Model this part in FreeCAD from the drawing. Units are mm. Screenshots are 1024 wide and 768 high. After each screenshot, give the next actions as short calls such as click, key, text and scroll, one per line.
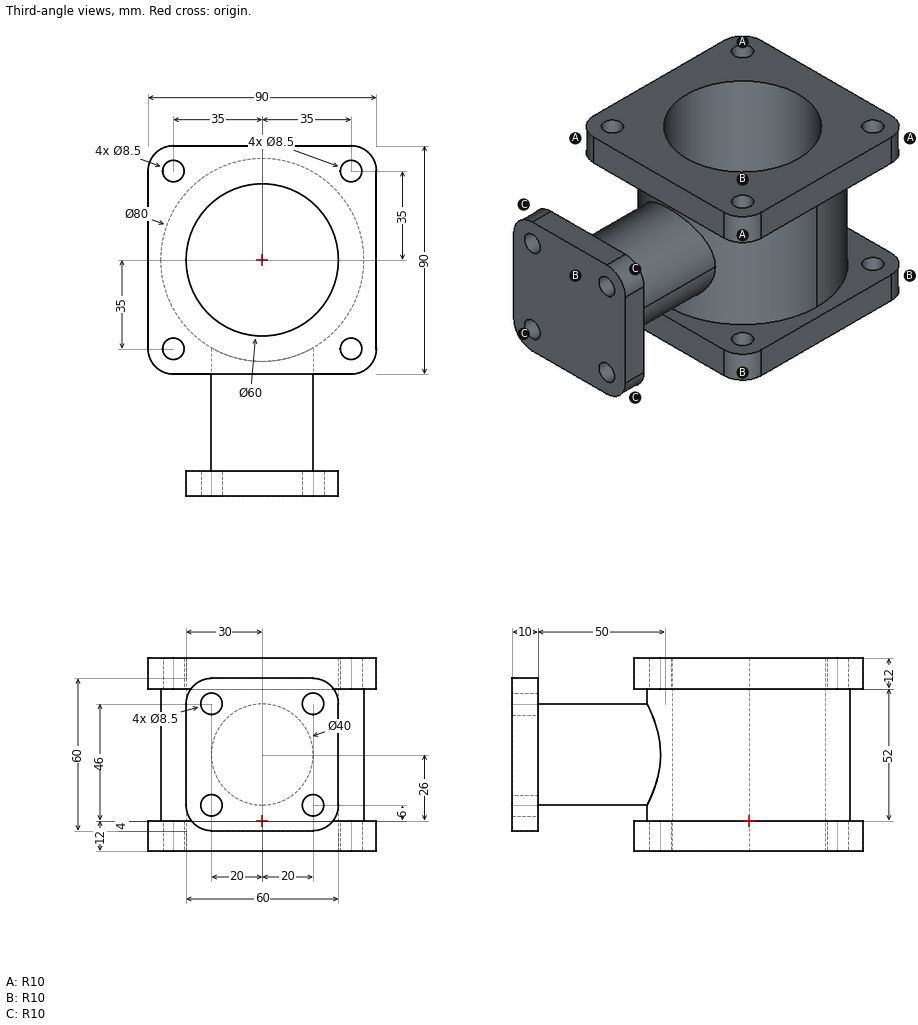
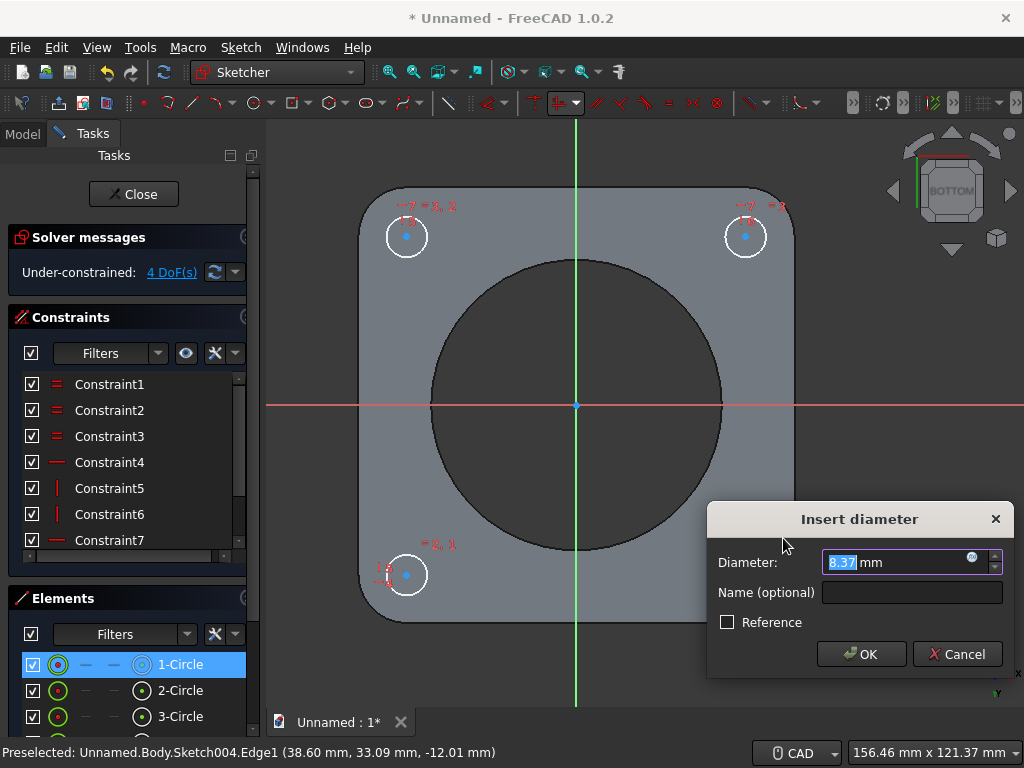
text(8.5)
key(Return)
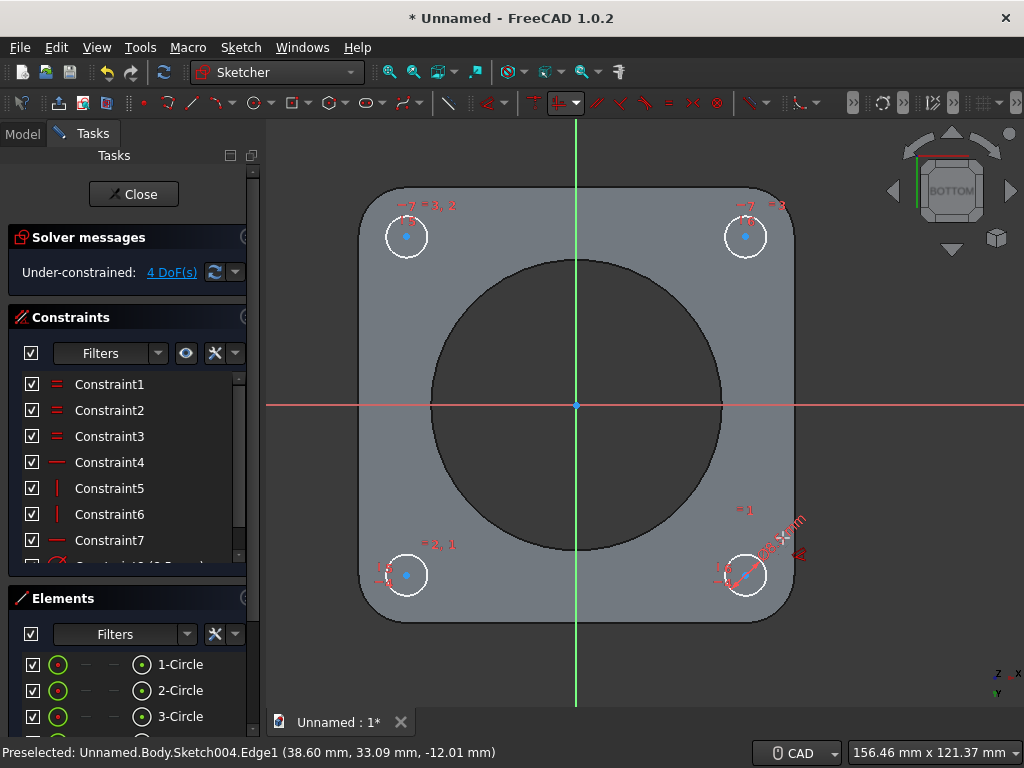
click(746, 575)
click(661, 609)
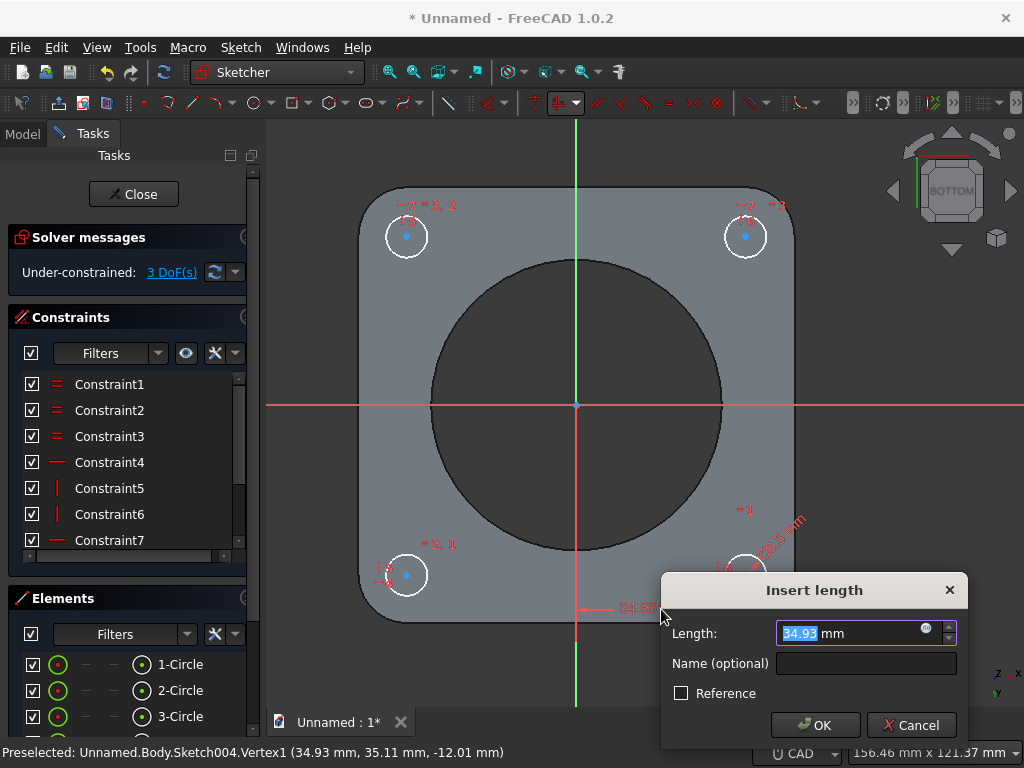
text(35)
key(Return)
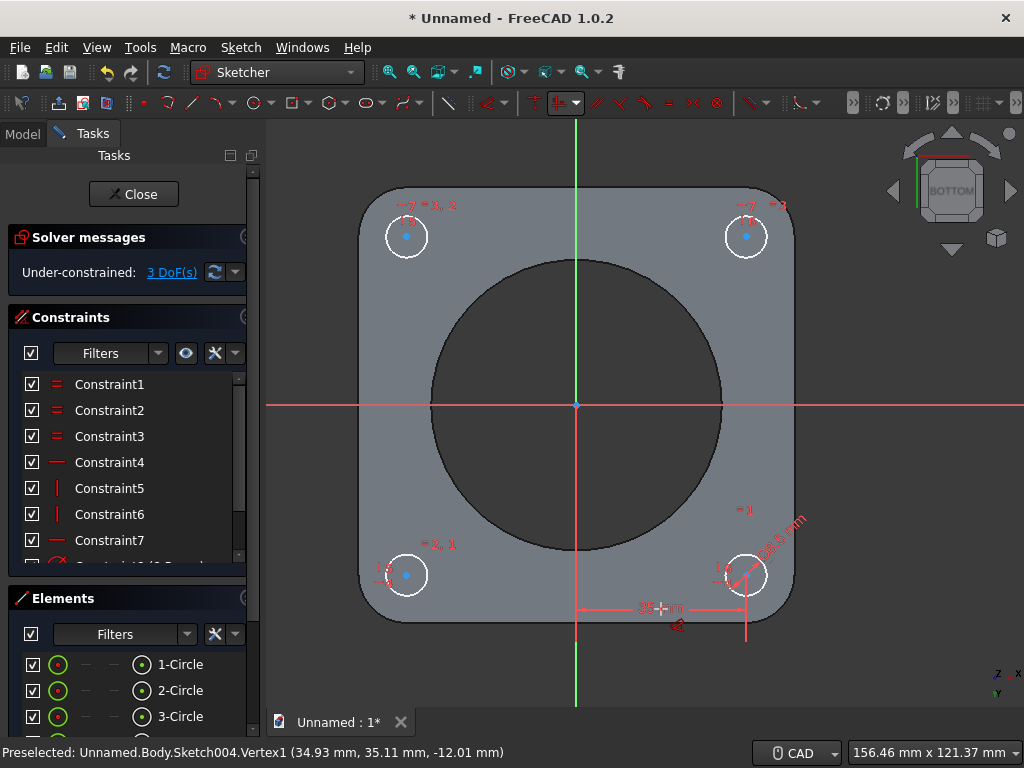
click(746, 575)
click(780, 490)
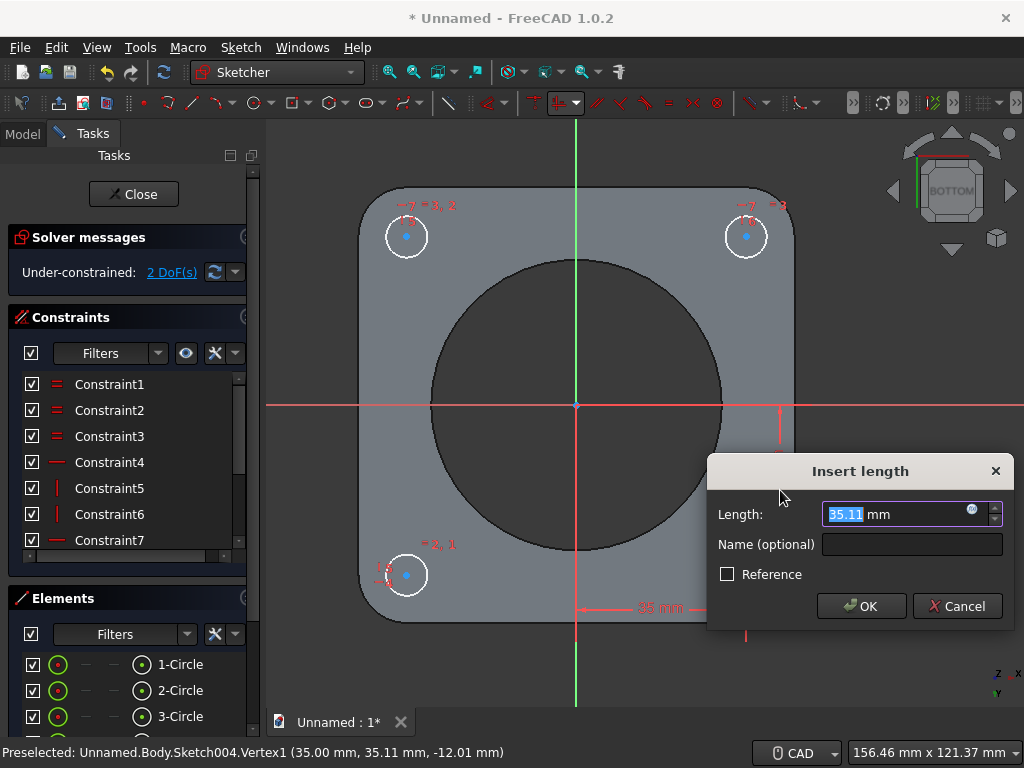
text(35)
key(Return)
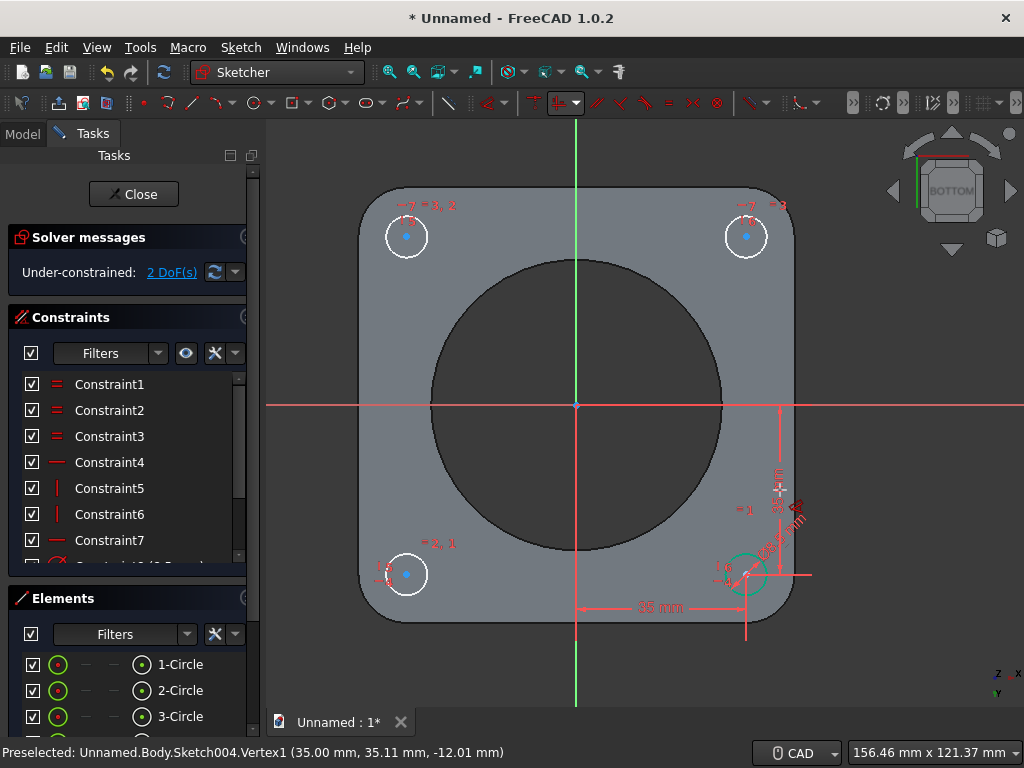
click(407, 575)
click(492, 609)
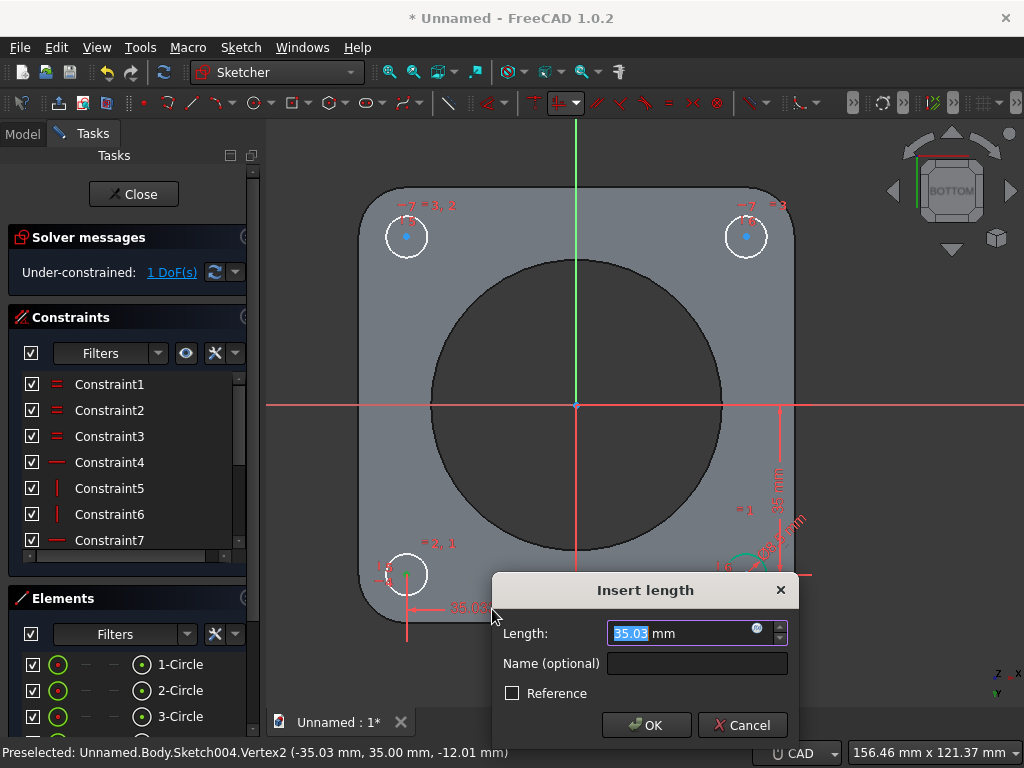
text(35)
key(Return)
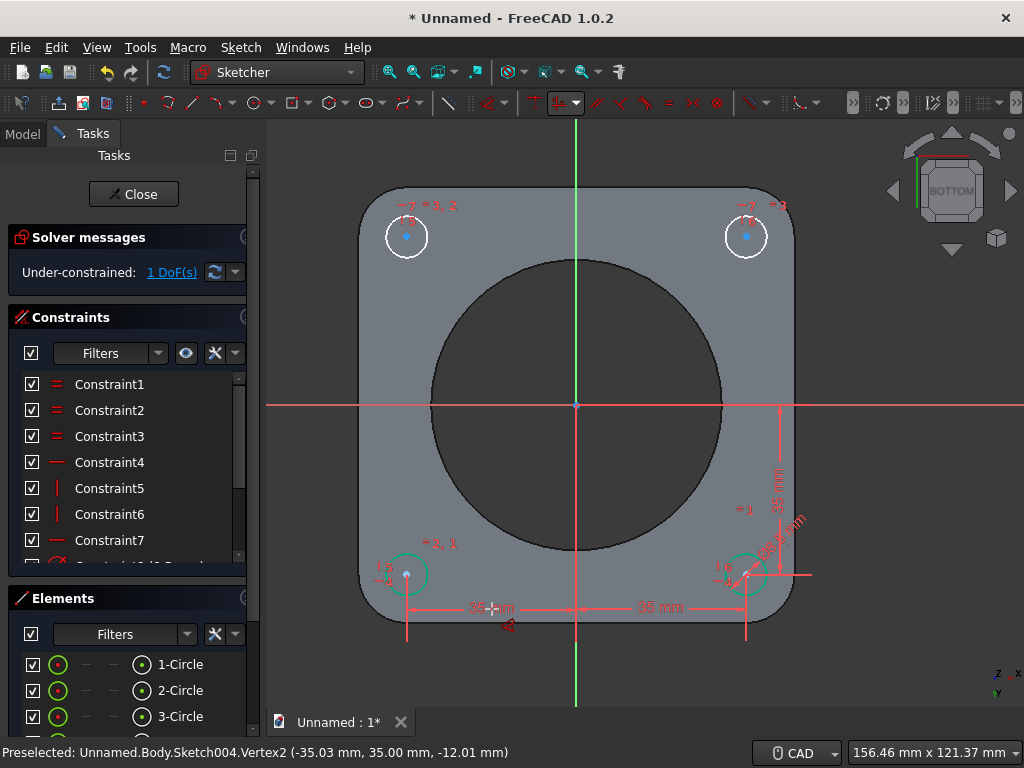
click(407, 237)
click(373, 321)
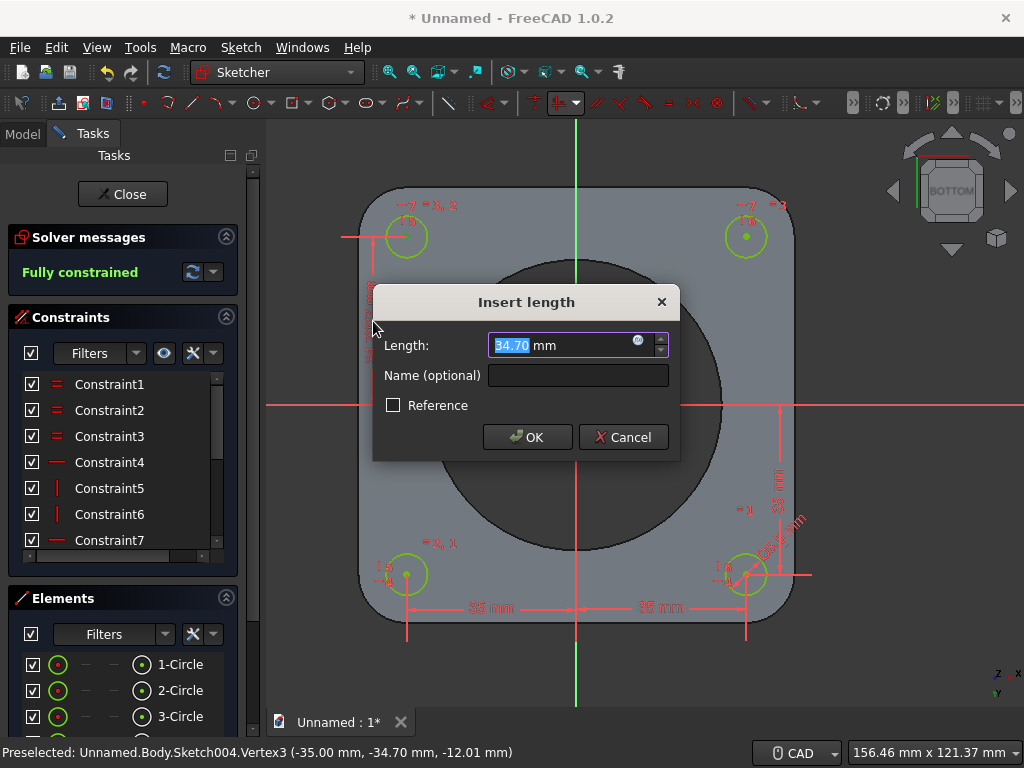
text(35)
key(Return)
key(Escape)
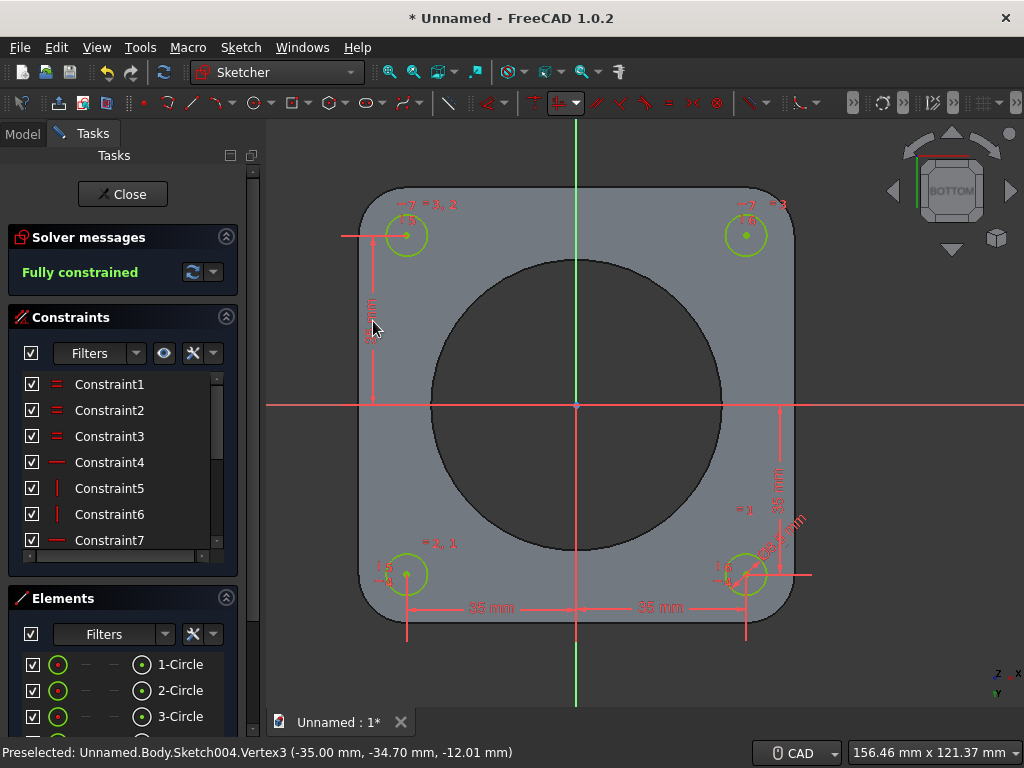
click(123, 194)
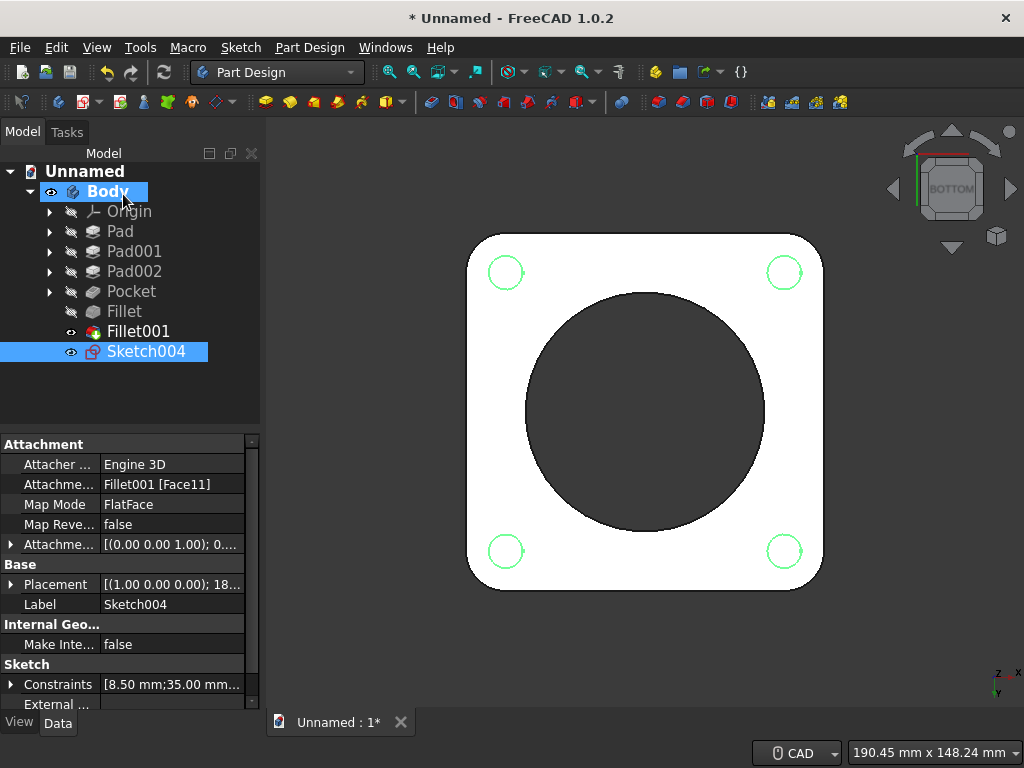
click(432, 102)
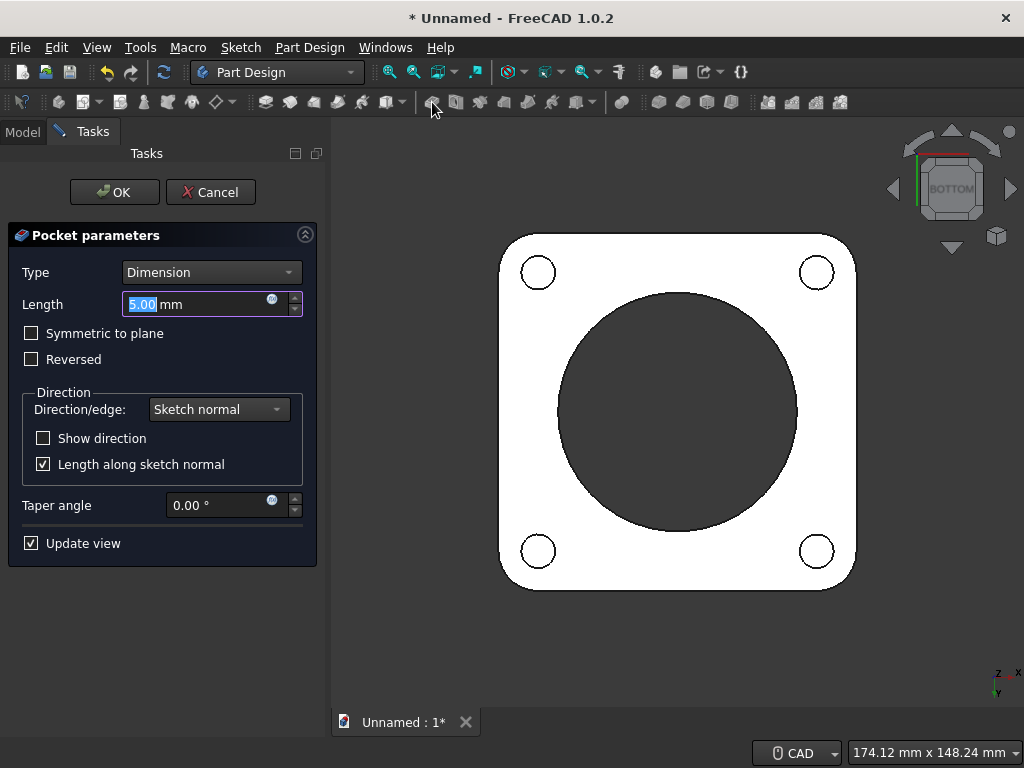
text(12)
key(Tab)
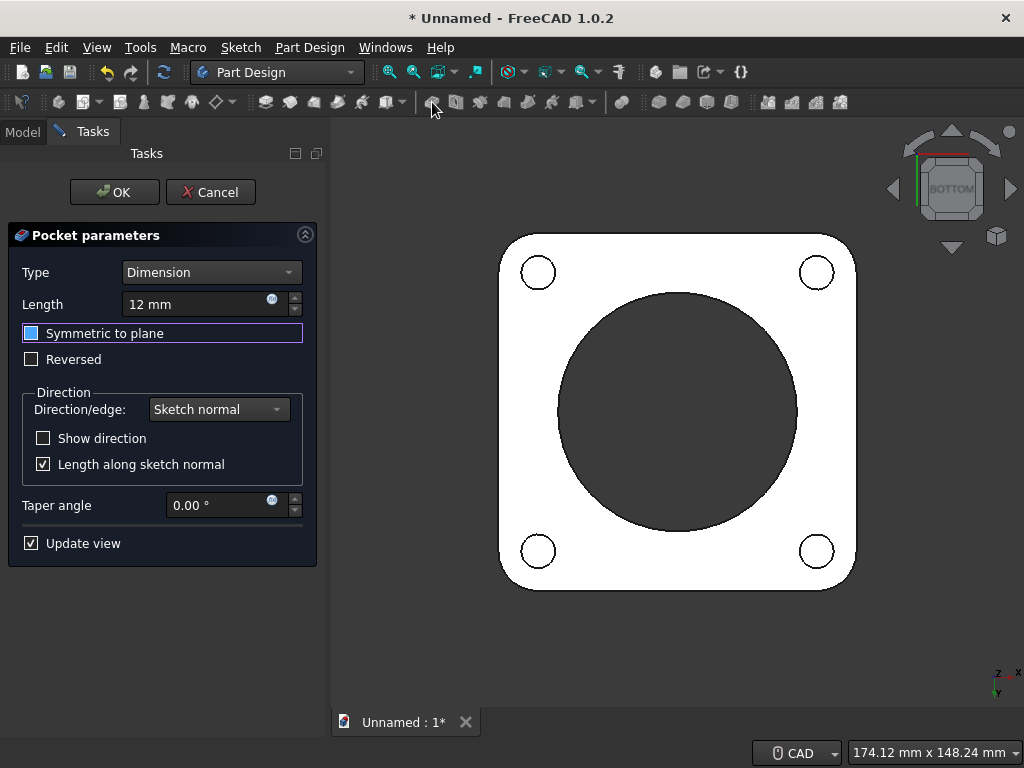
click(115, 192)